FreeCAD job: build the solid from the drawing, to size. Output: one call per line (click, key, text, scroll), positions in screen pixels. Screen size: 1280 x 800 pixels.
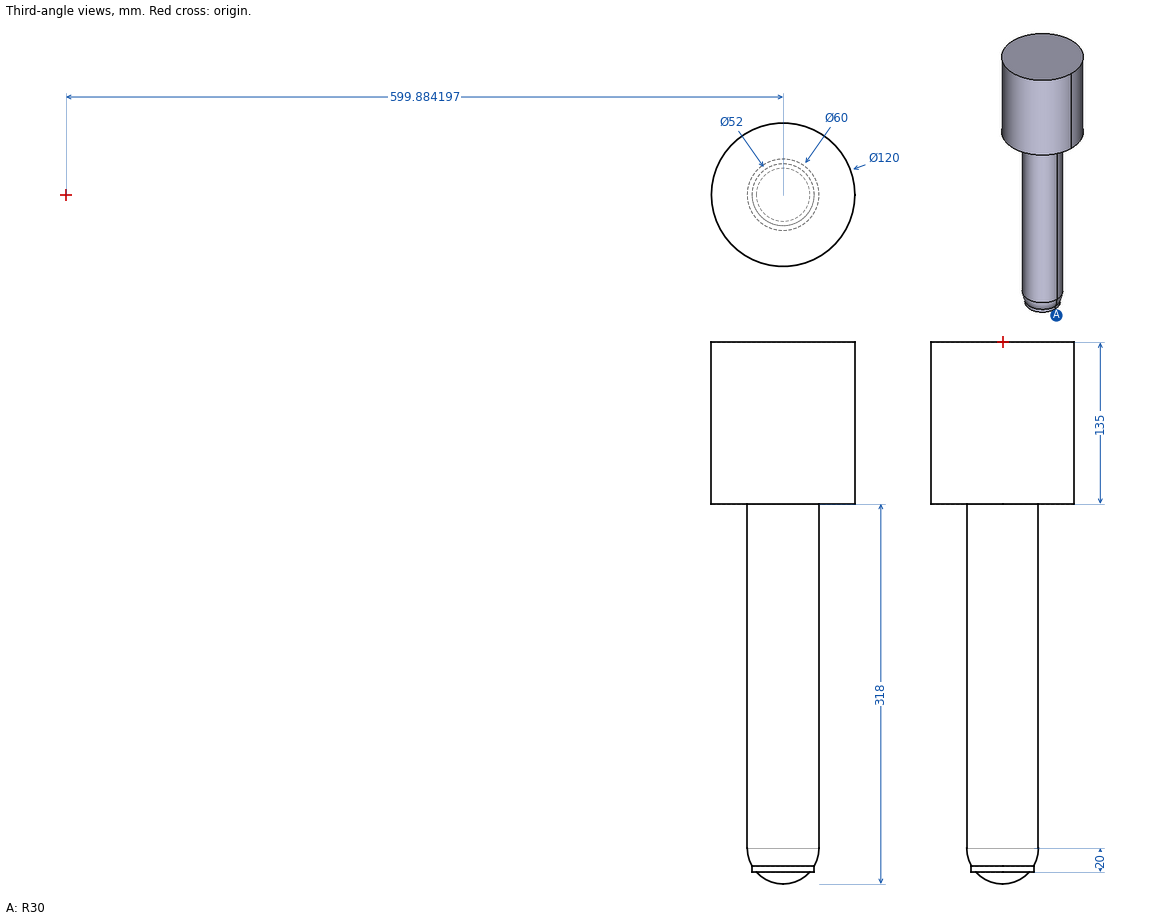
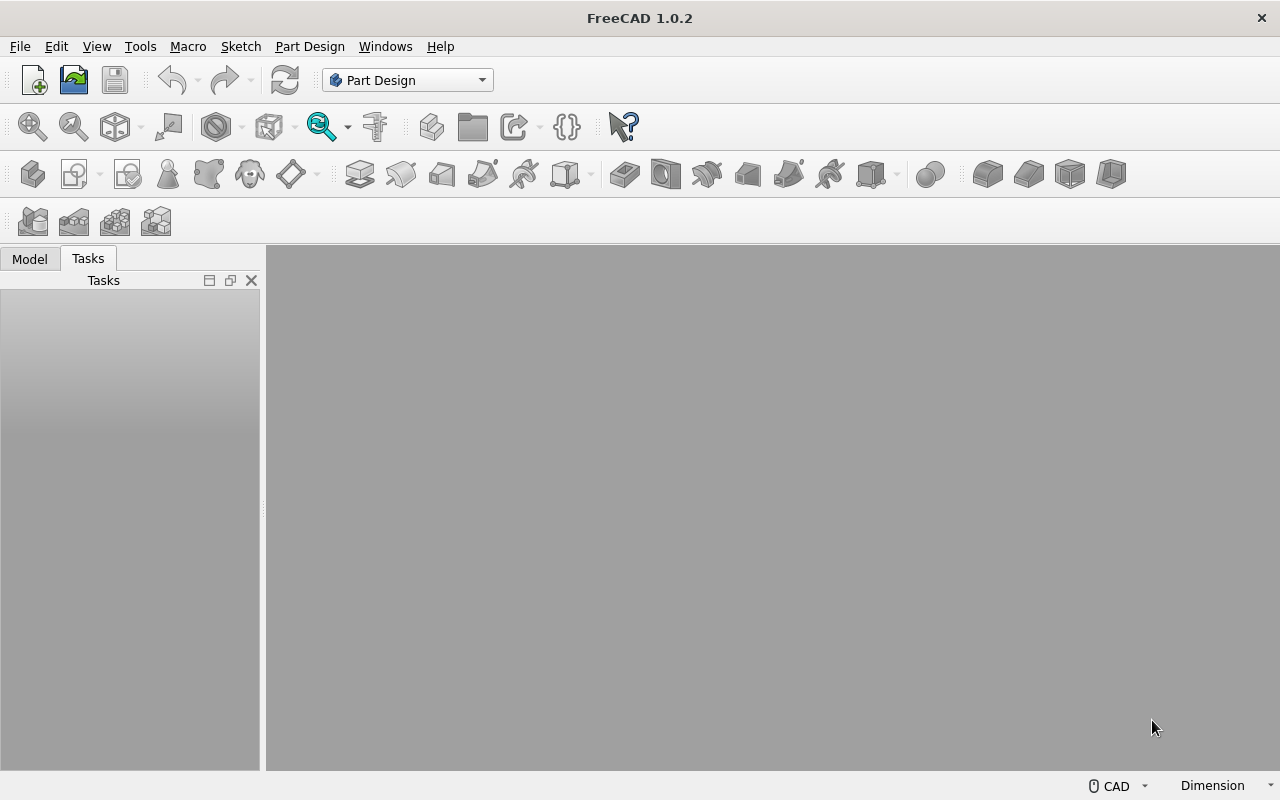
click(33, 80)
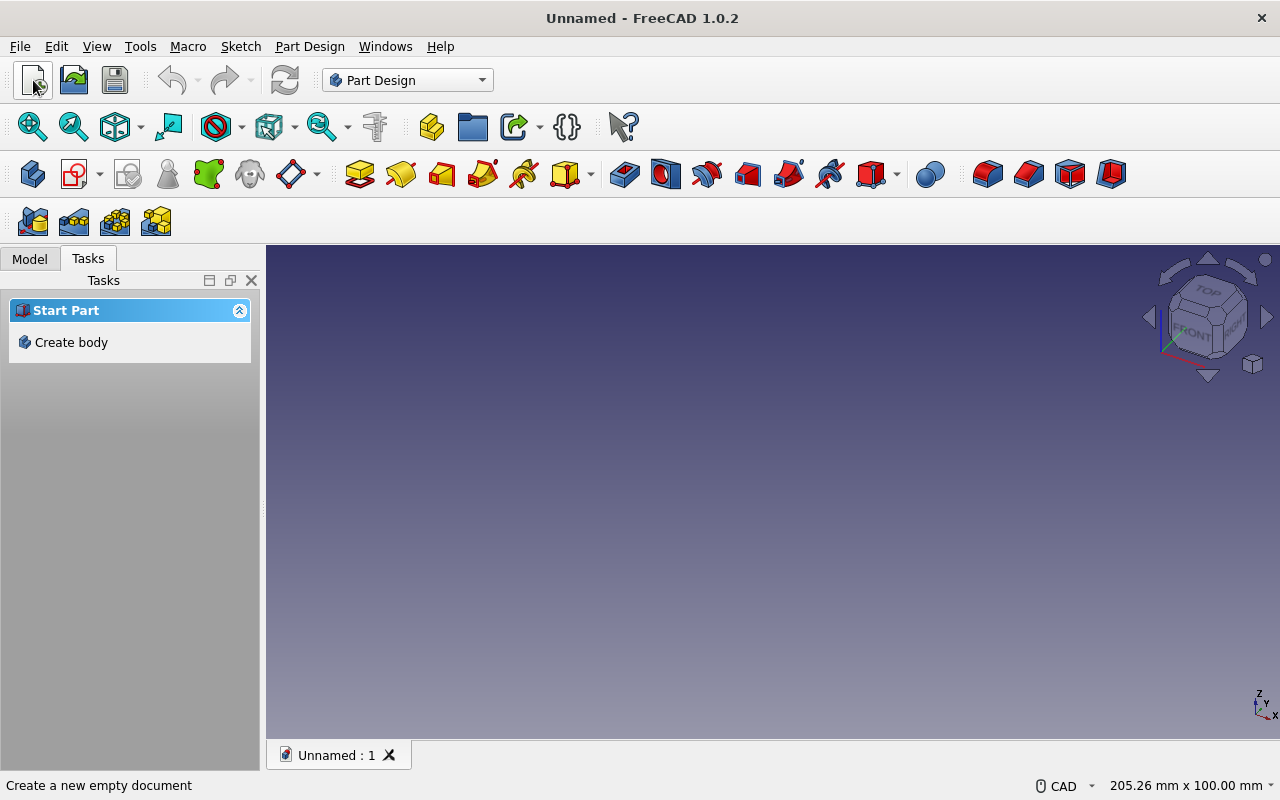
click(74, 174)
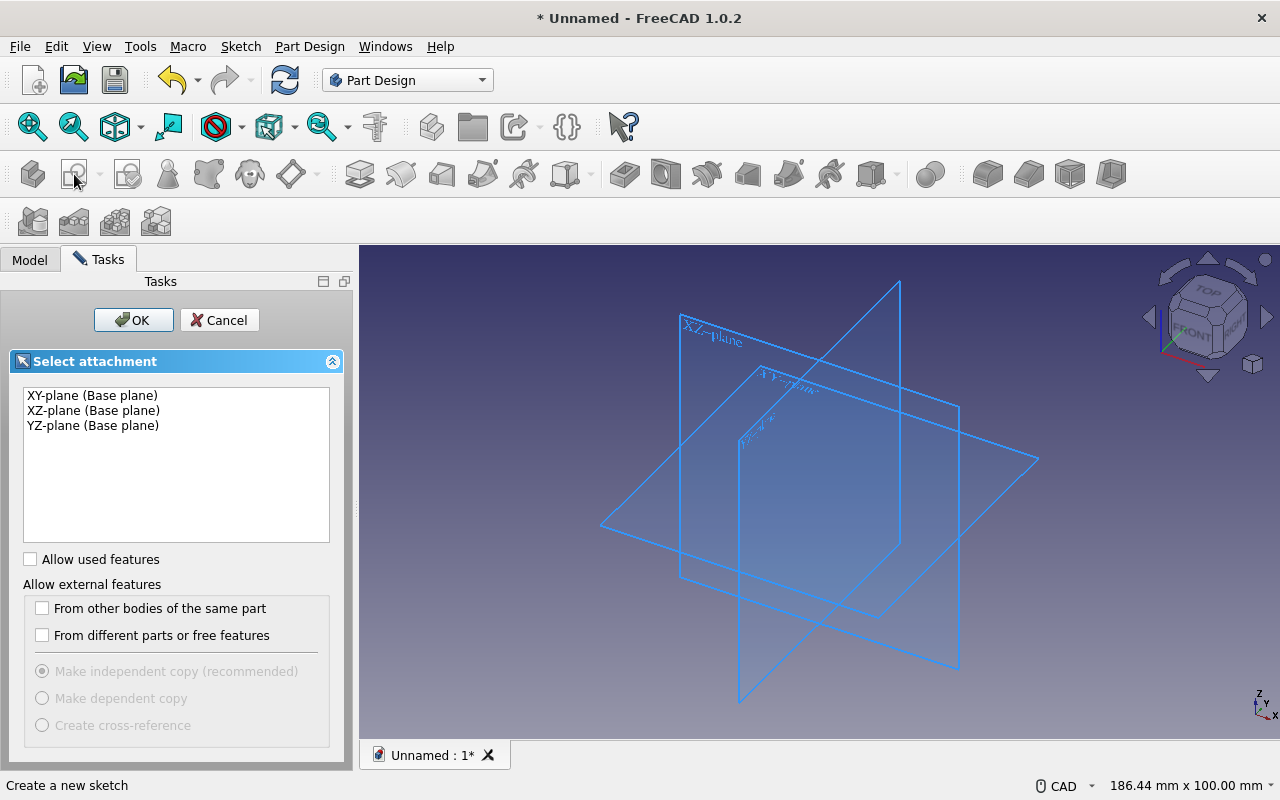
click(84, 396)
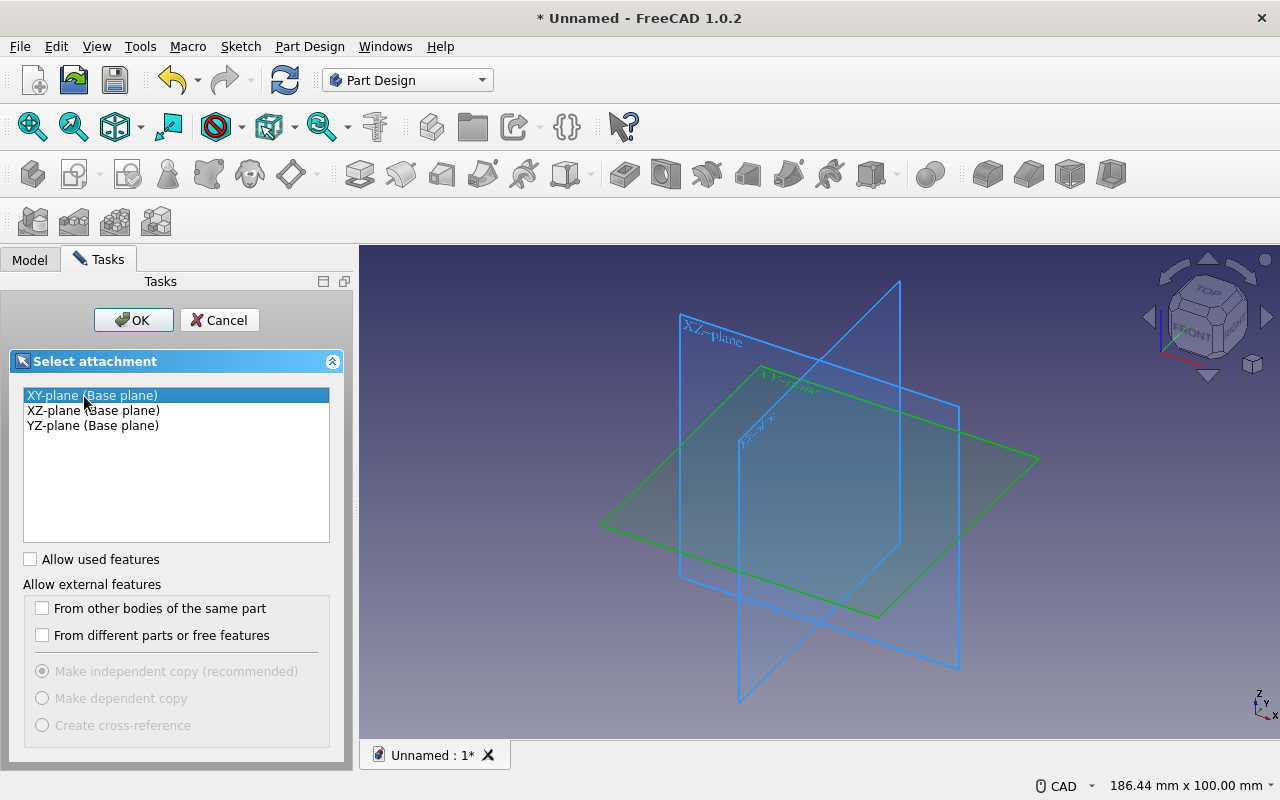
click(134, 320)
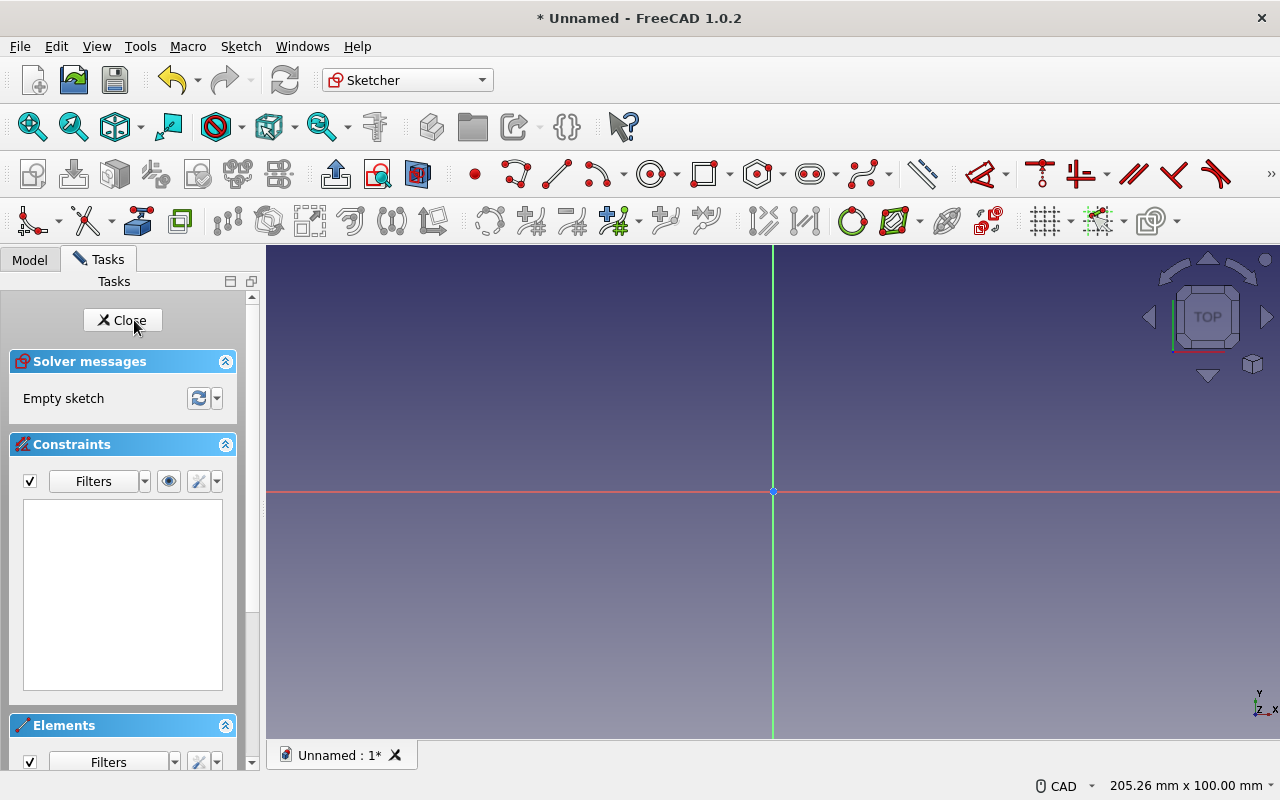
scroll(704, 492, down, 5)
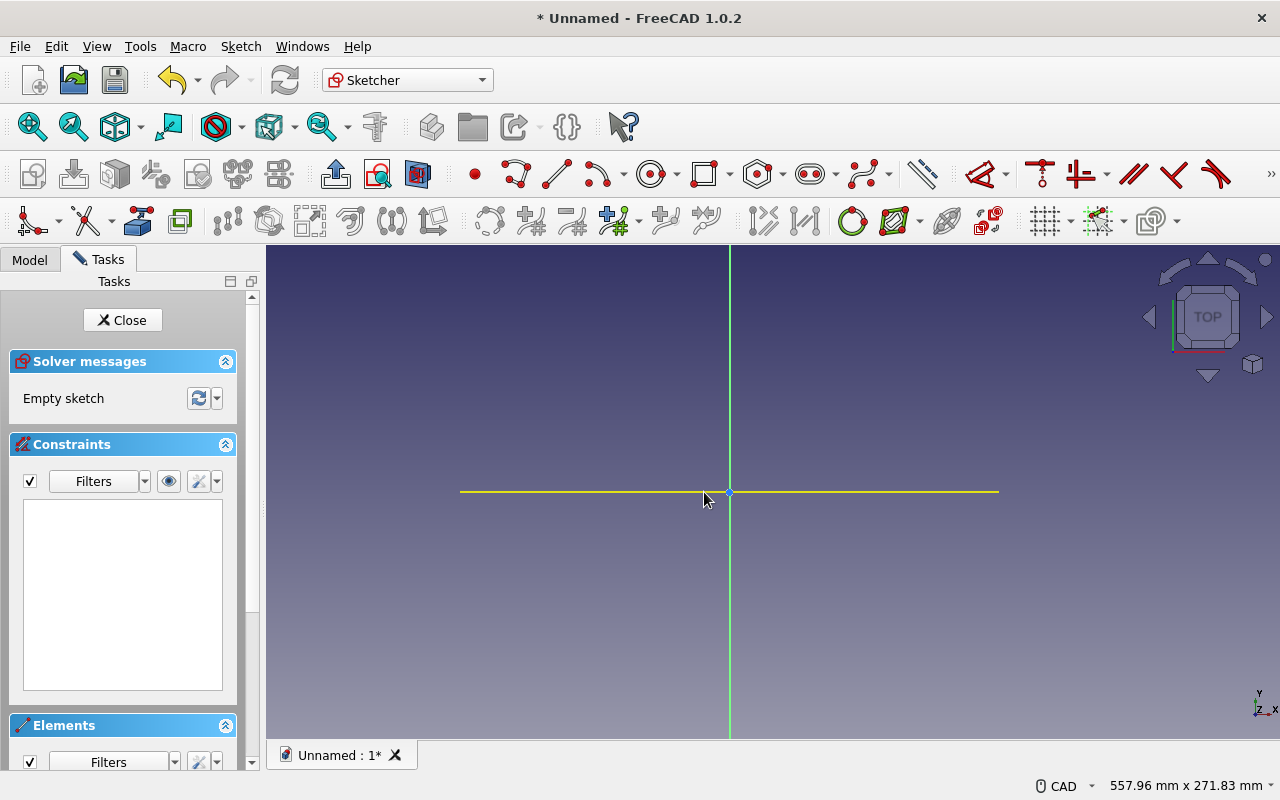
scroll(704, 492, down, 5)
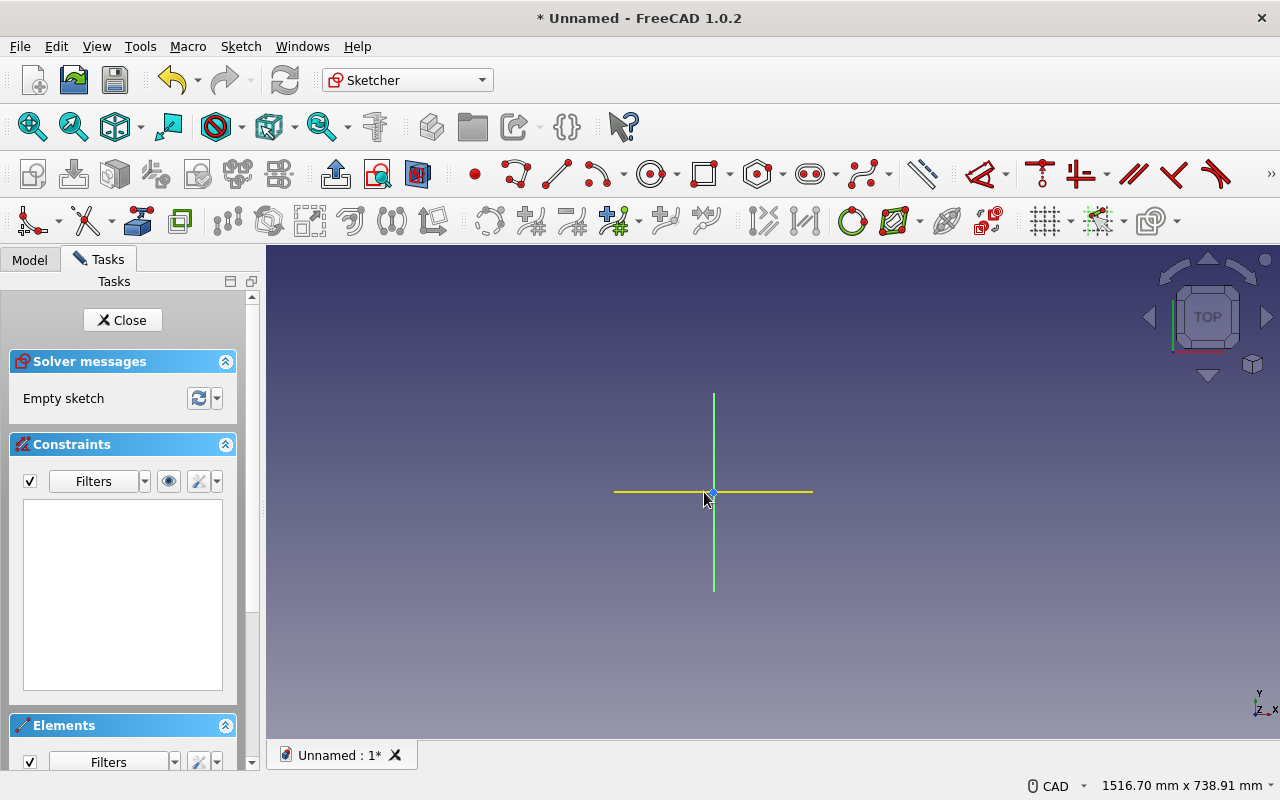
scroll(704, 492, down, 5)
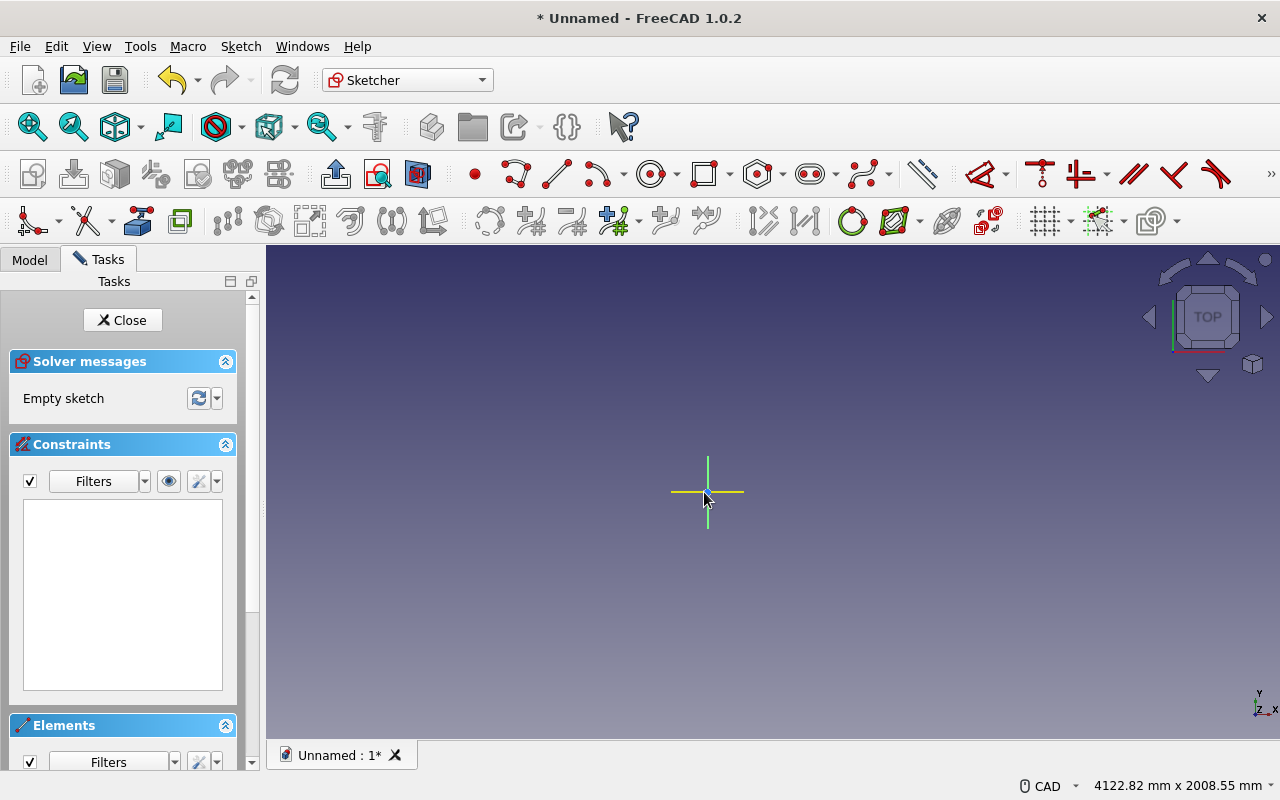
scroll(870, 493, up, 12)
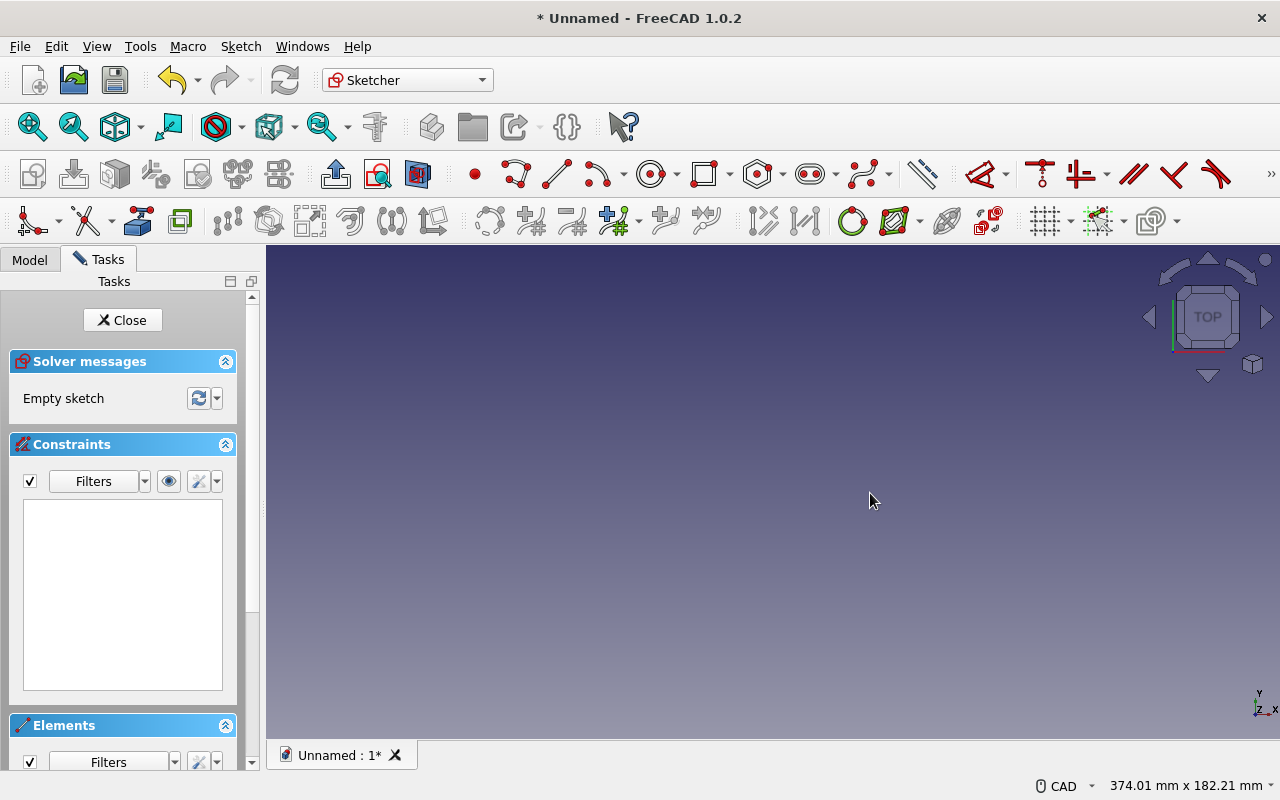
click(650, 174)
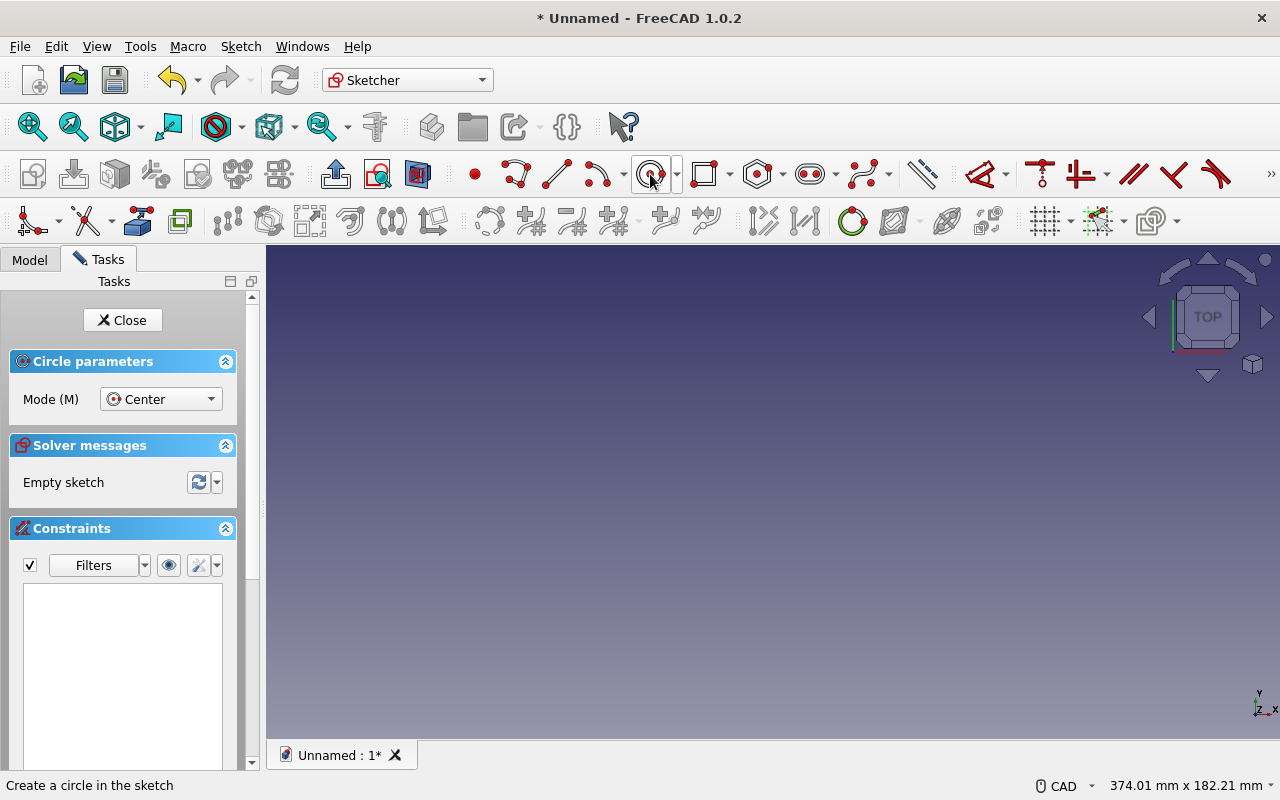
click(703, 482)
move(818, 367)